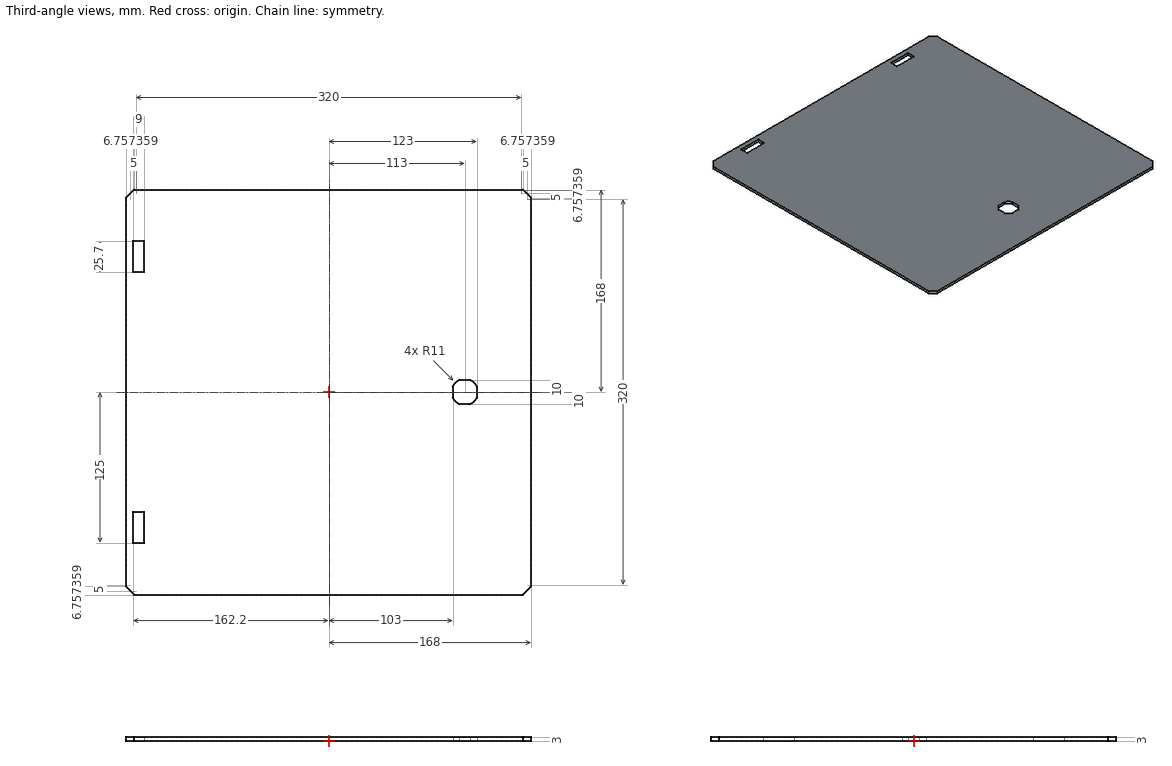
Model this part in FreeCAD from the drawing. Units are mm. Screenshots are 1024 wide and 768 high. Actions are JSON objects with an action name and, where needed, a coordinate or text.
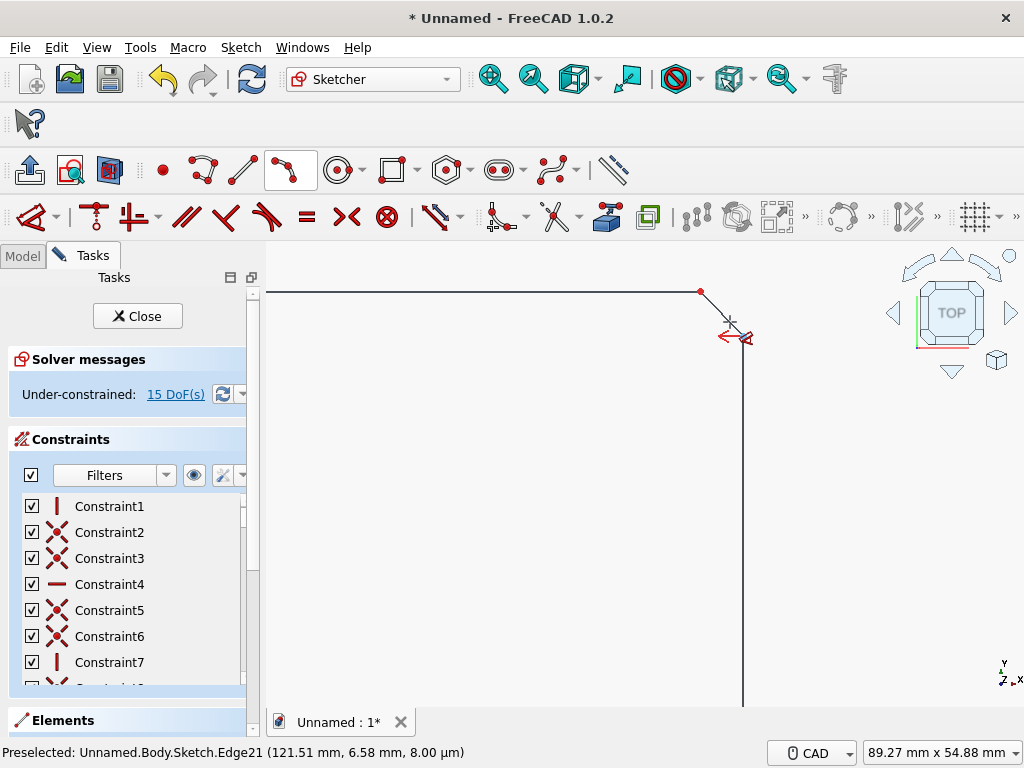
{"action": "left_click", "coordinate": [726, 319]}
{"action": "left_click", "coordinate": [722, 370]}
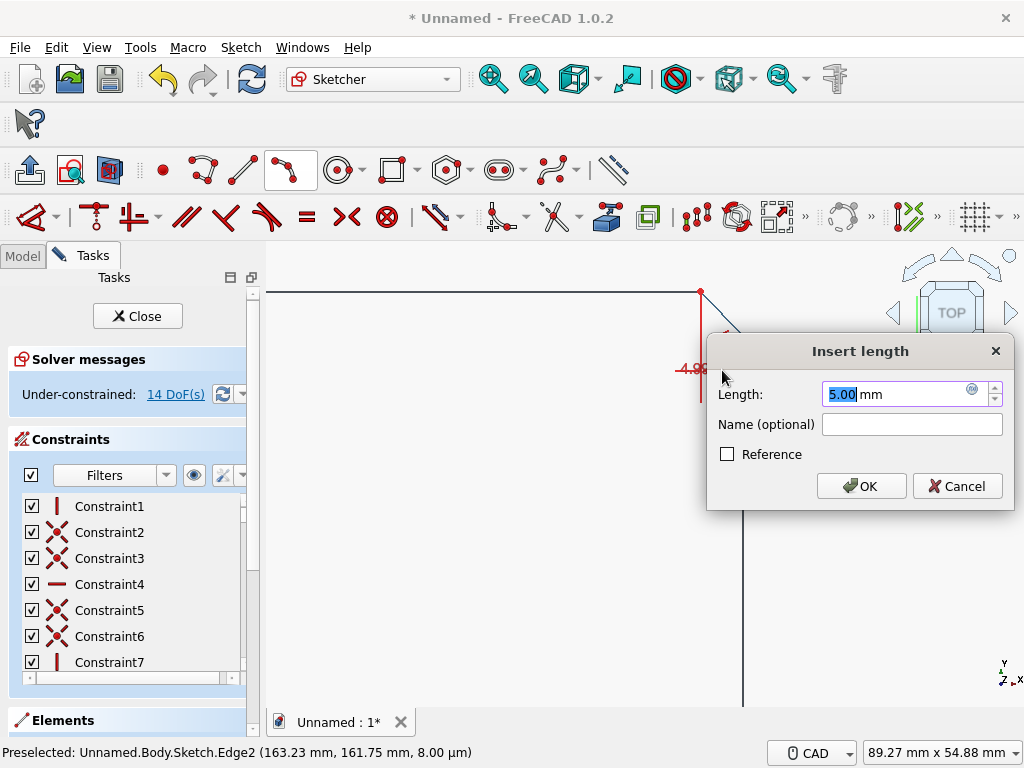
{"action": "type", "text": "5"}
{"action": "key", "text": "Return"}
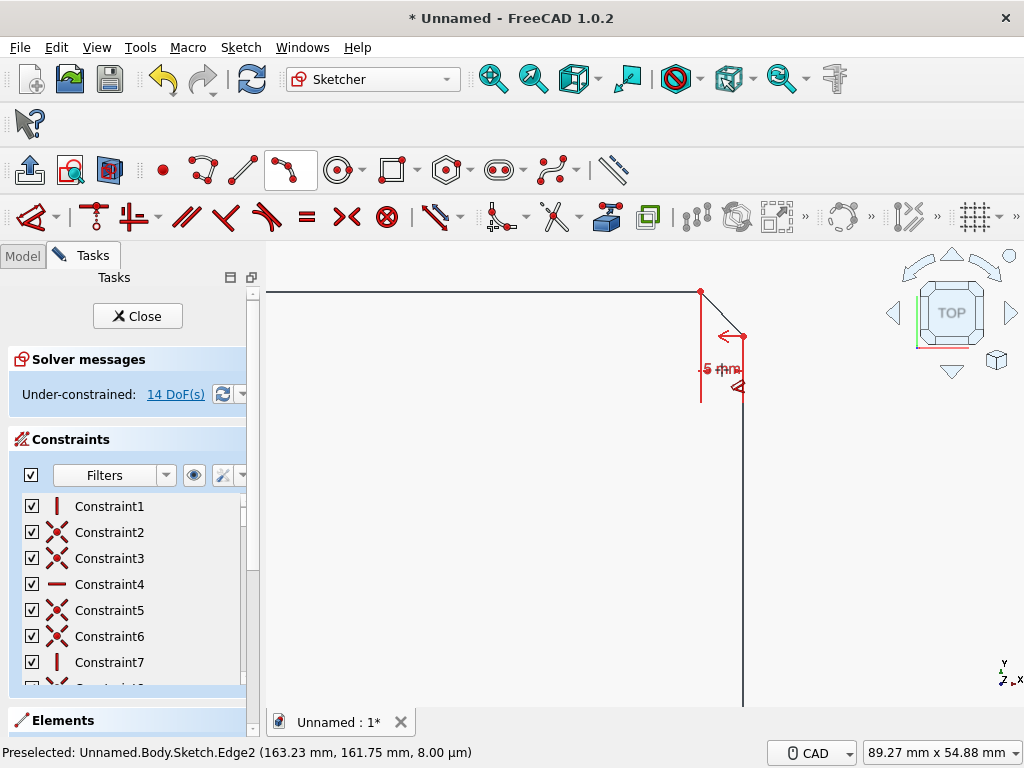
{"action": "left_click", "coordinate": [731, 323]}
{"action": "left_click", "coordinate": [777, 314]}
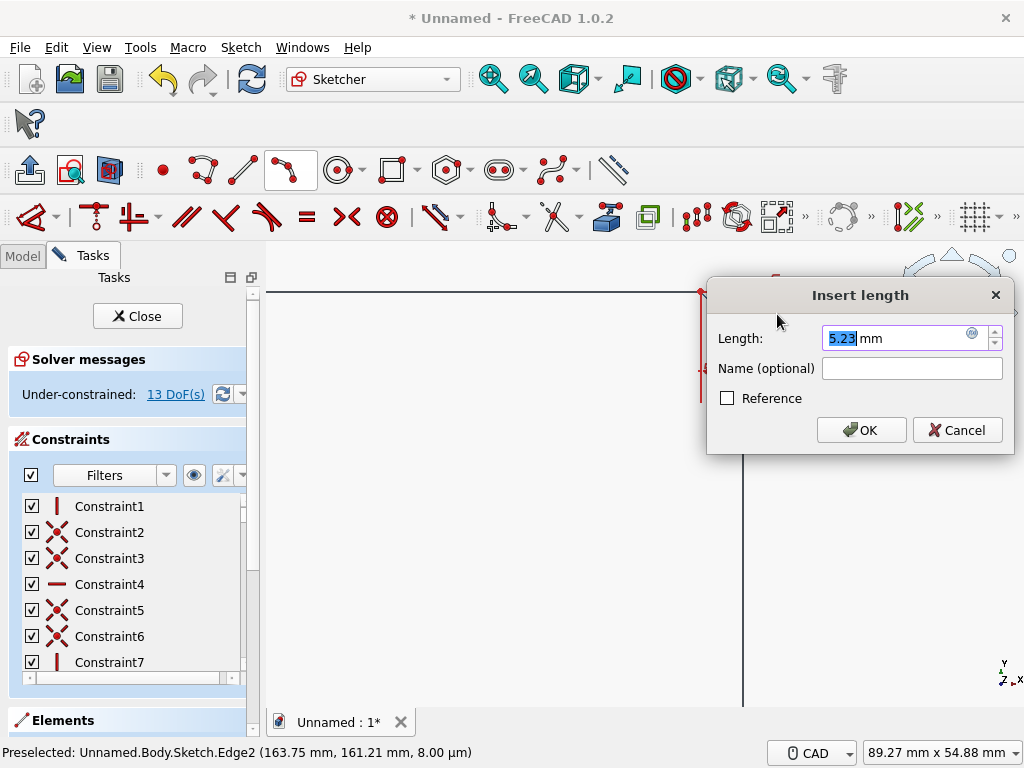
{"action": "type", "text": "5"}
{"action": "key", "text": "Return"}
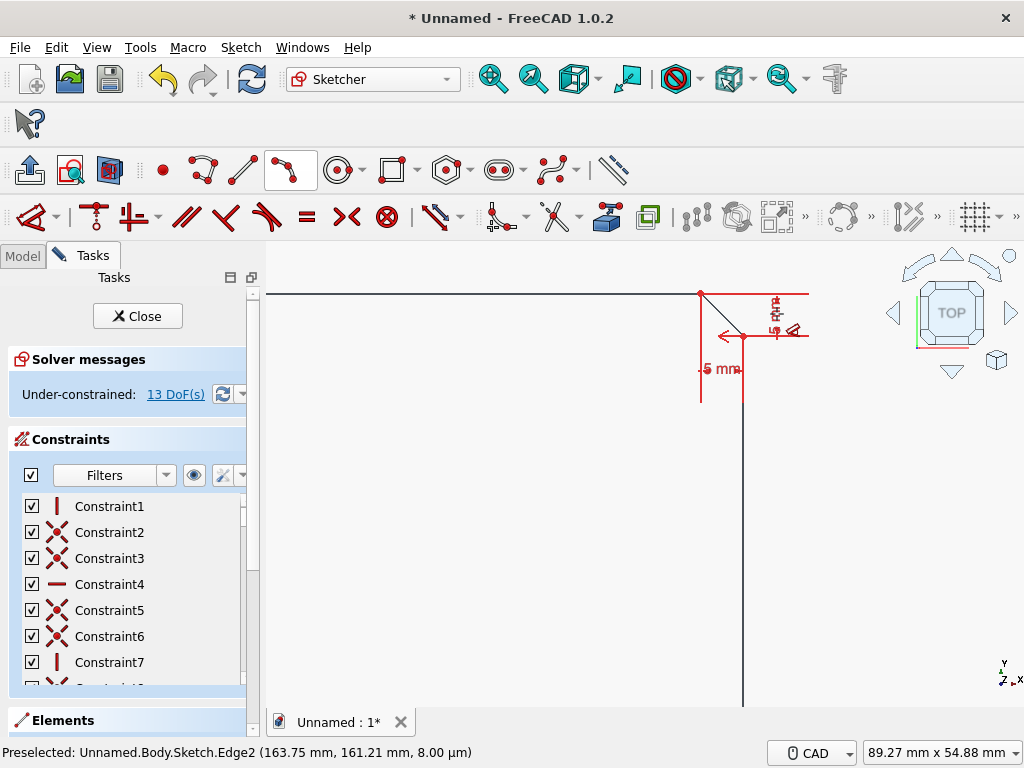
{"action": "scroll", "coordinate": [730, 322], "scroll_direction": "down", "scroll_amount": 11}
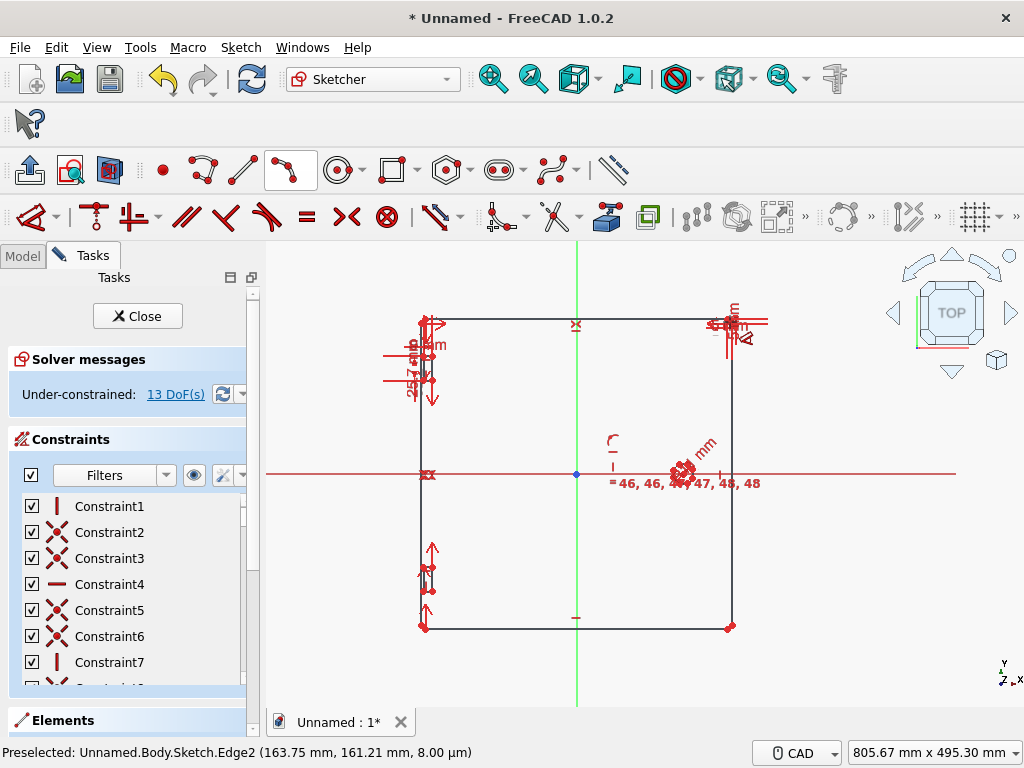
{"action": "scroll", "coordinate": [424, 320], "scroll_direction": "up", "scroll_amount": 11}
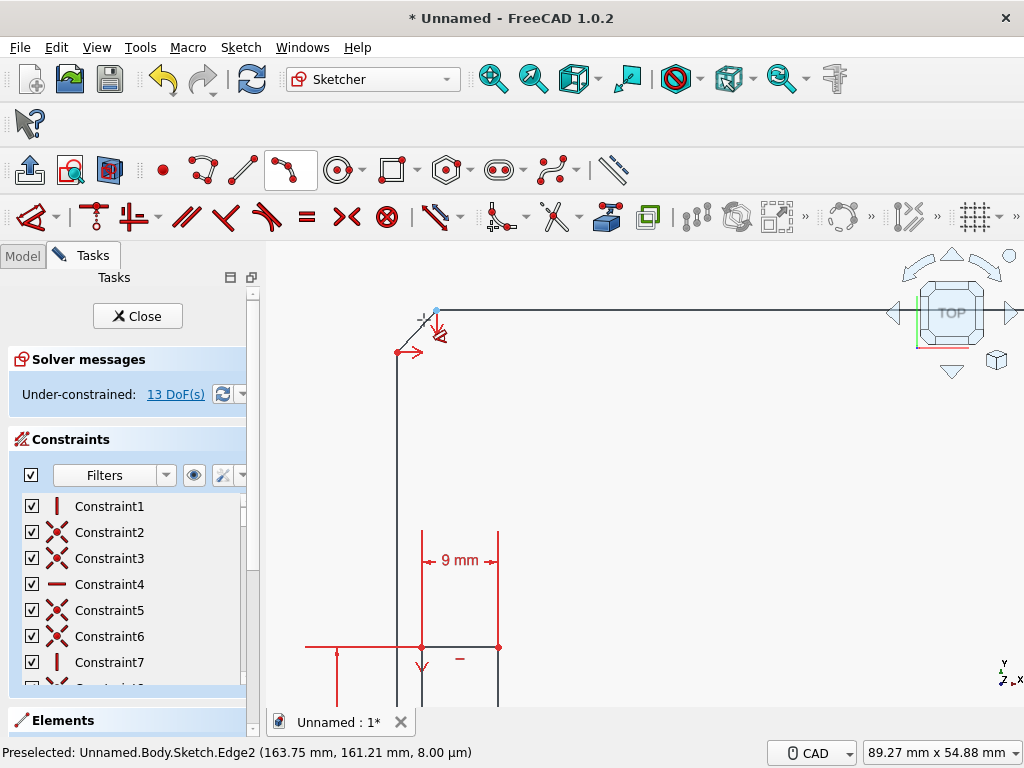
{"action": "left_click", "coordinate": [425, 323]}
{"action": "left_click", "coordinate": [417, 276]}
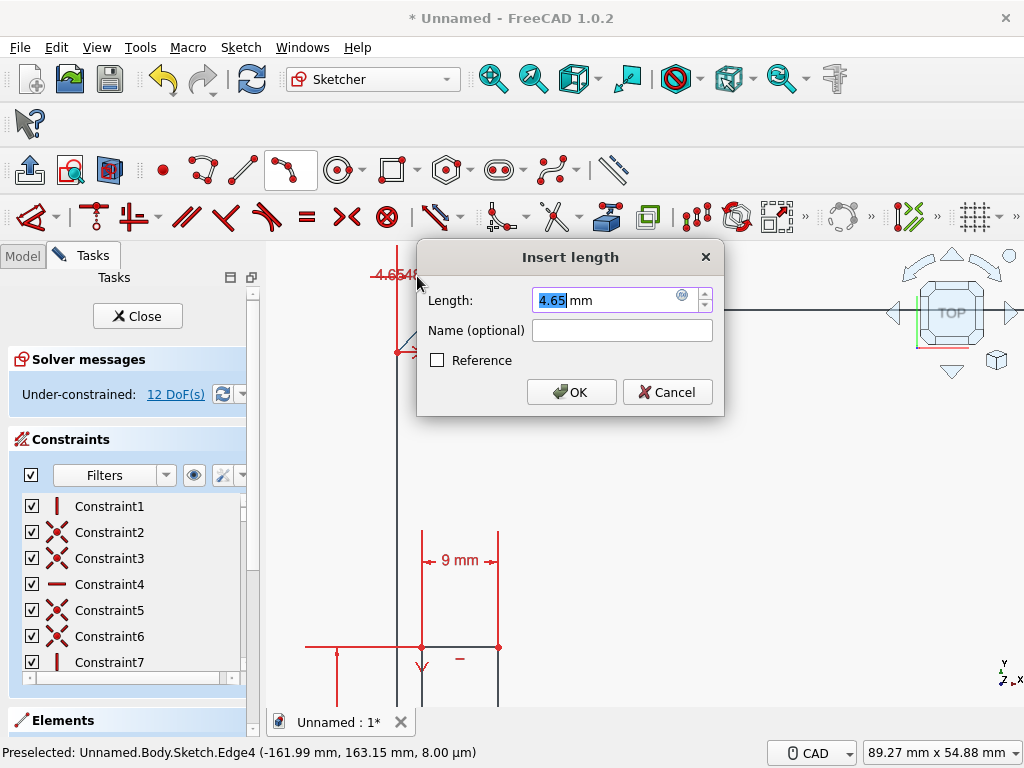
{"action": "type", "text": "5"}
{"action": "key", "text": "Return"}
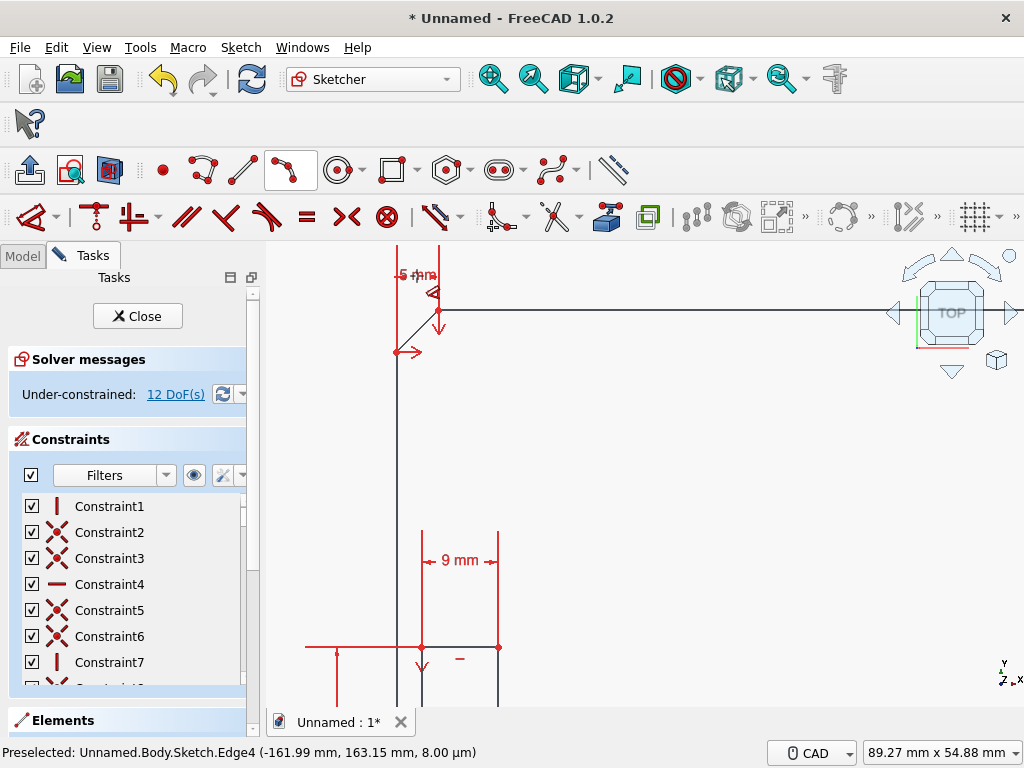
{"action": "scroll", "coordinate": [424, 320], "scroll_direction": "down", "scroll_amount": 11}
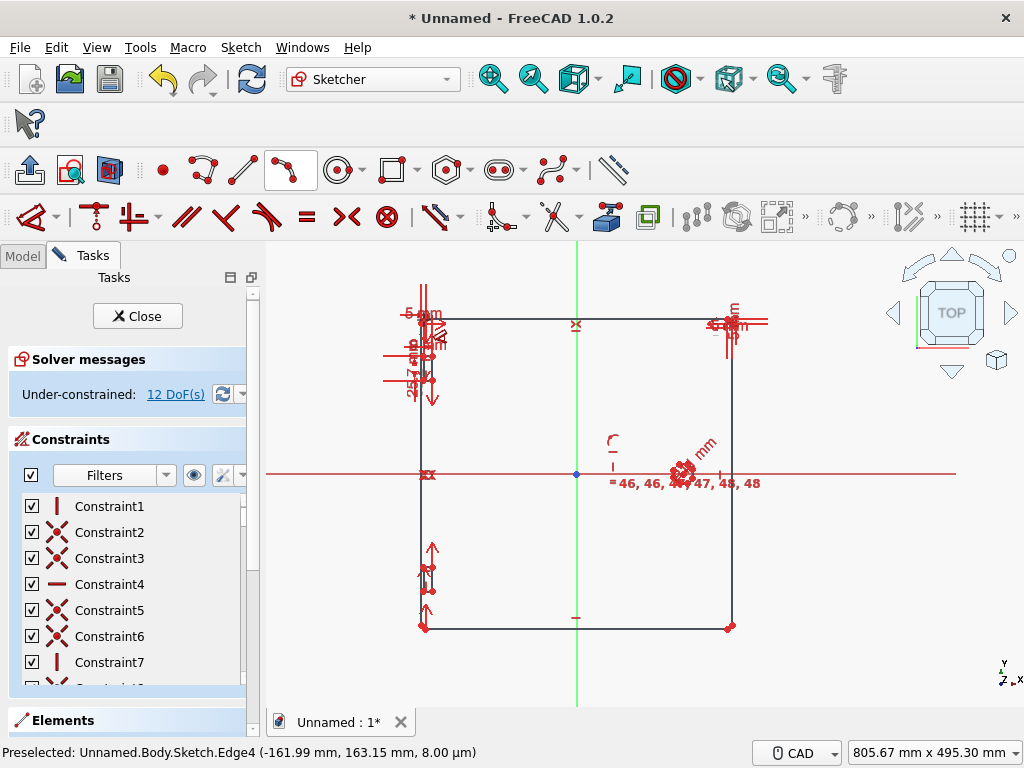
{"action": "scroll", "coordinate": [423, 627], "scroll_direction": "up", "scroll_amount": 11}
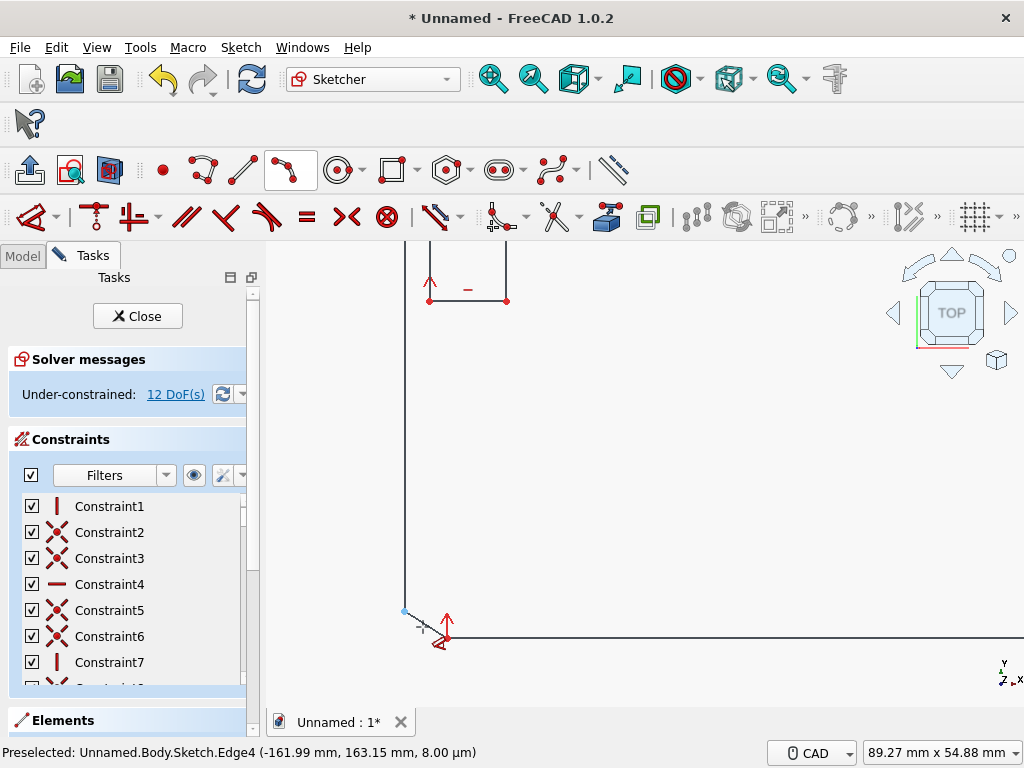
{"action": "left_click", "coordinate": [417, 619]}
{"action": "left_click", "coordinate": [371, 625]}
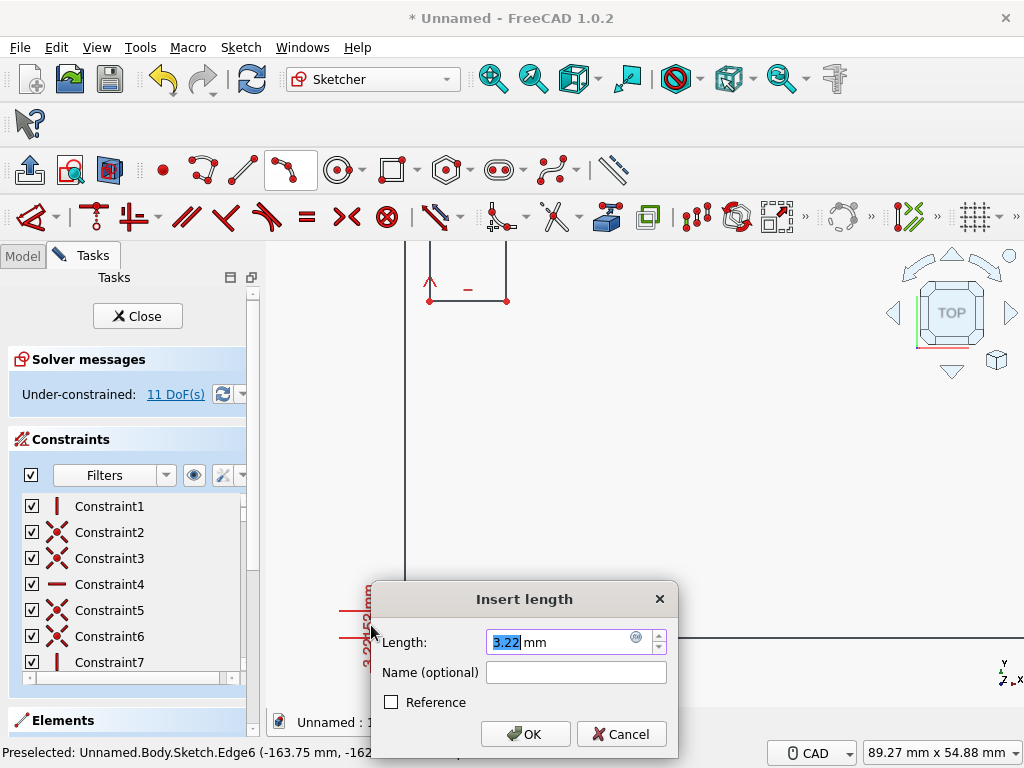
{"action": "type", "text": "5"}
{"action": "key", "text": "Return"}